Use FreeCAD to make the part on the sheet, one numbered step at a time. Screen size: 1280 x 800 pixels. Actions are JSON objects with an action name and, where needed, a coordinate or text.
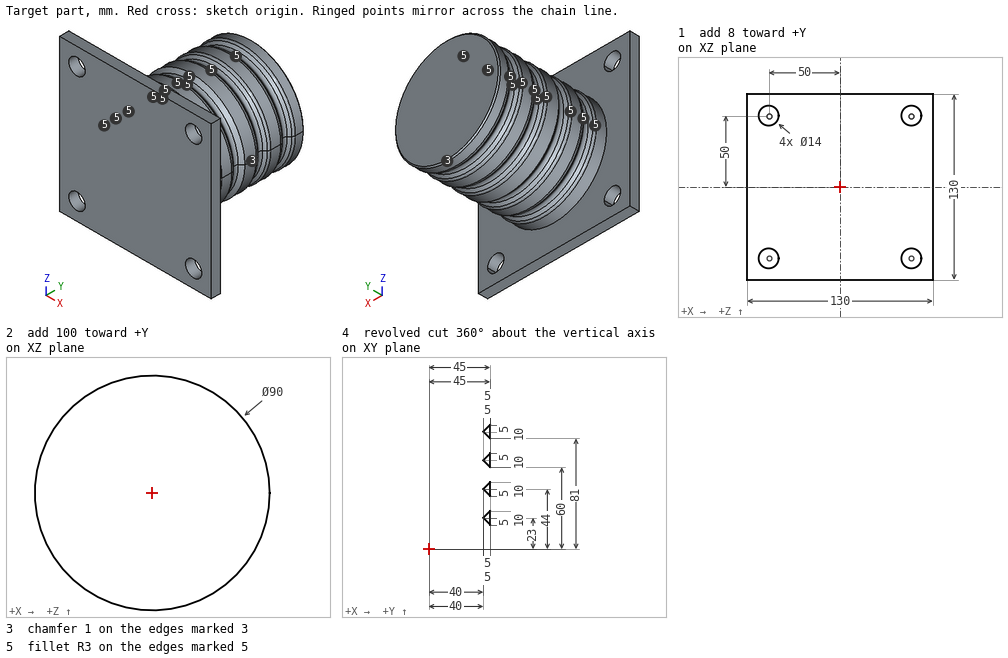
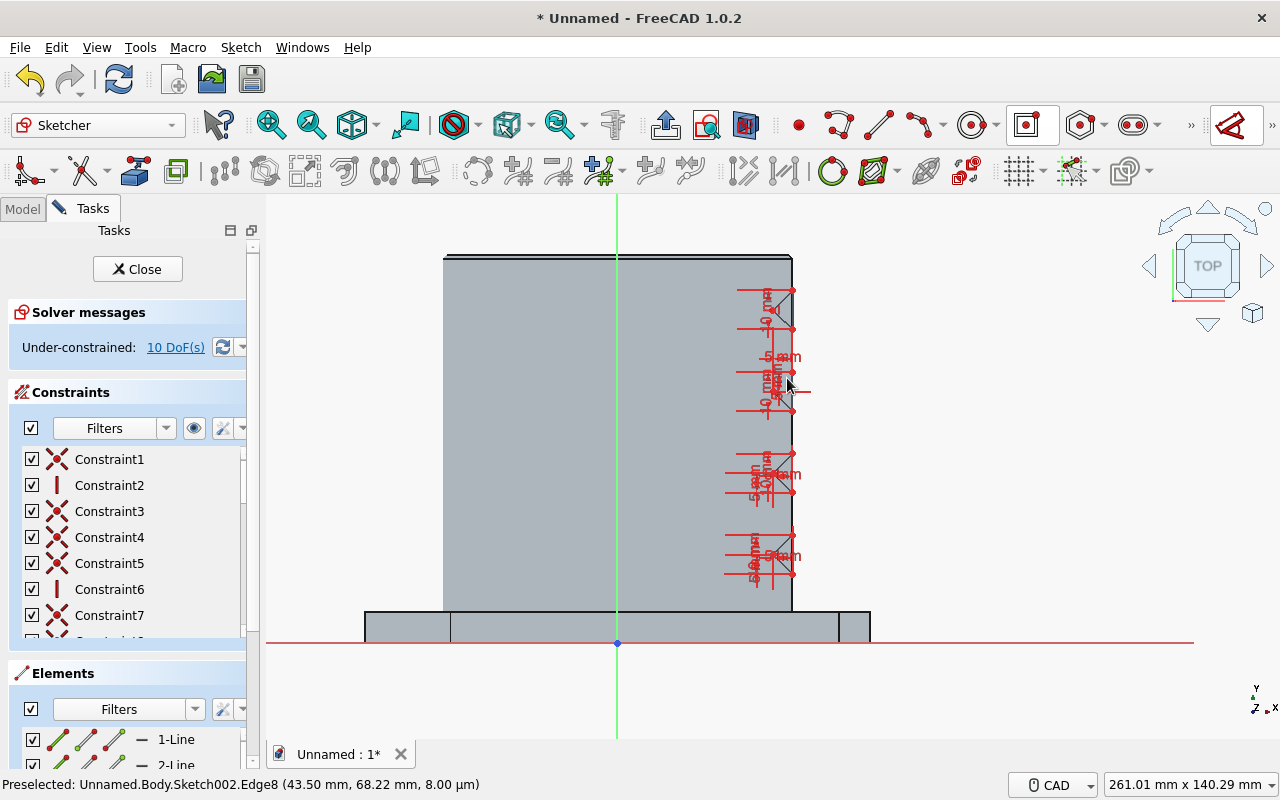
{"action": "scroll", "coordinate": [787, 296], "scroll_direction": "up", "scroll_amount": 5}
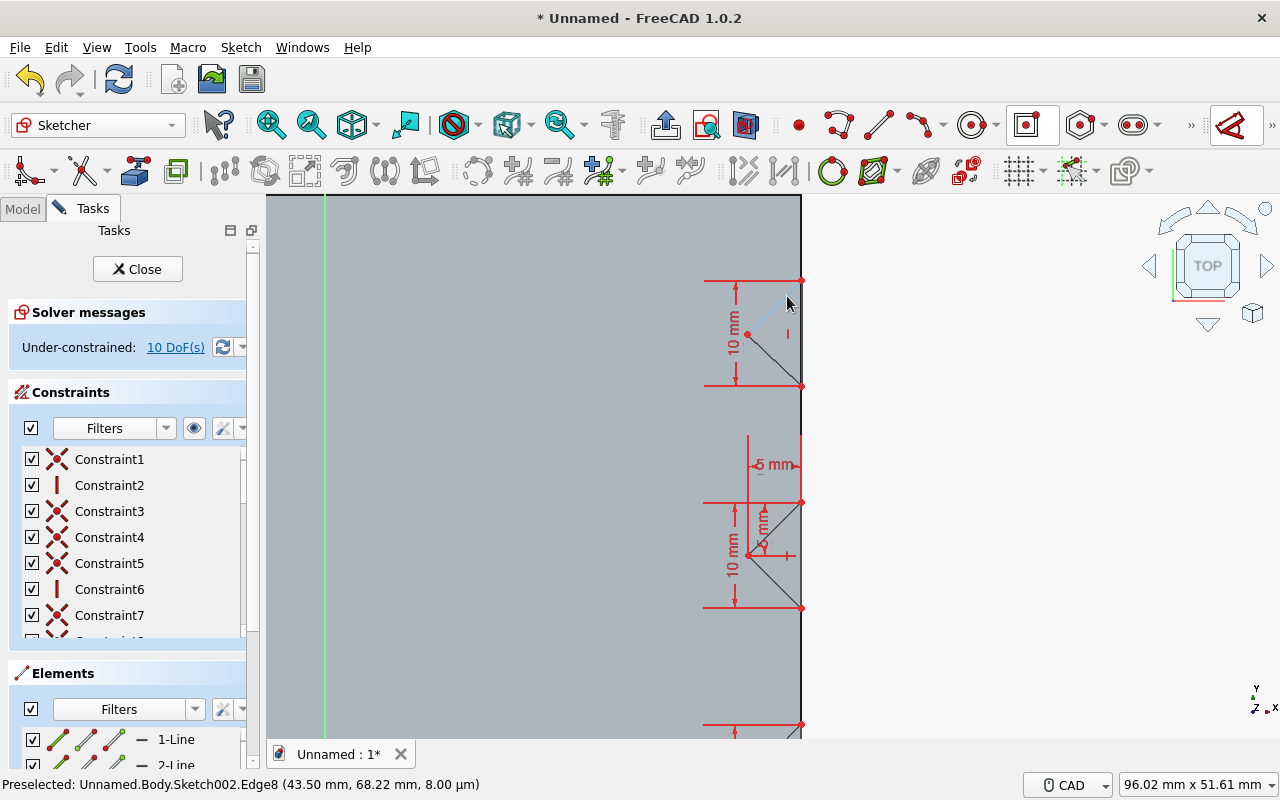
{"action": "left_click", "coordinate": [786, 297]}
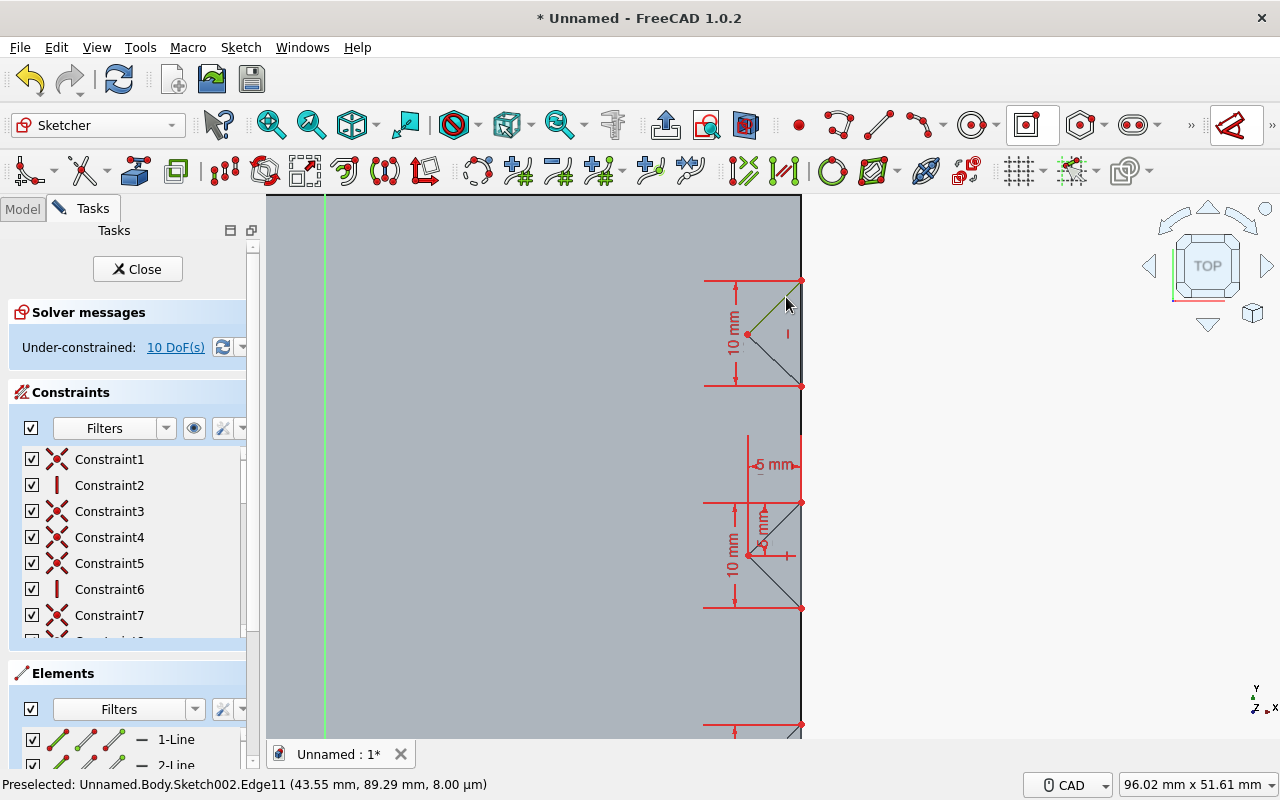
{"action": "key", "text": "l"}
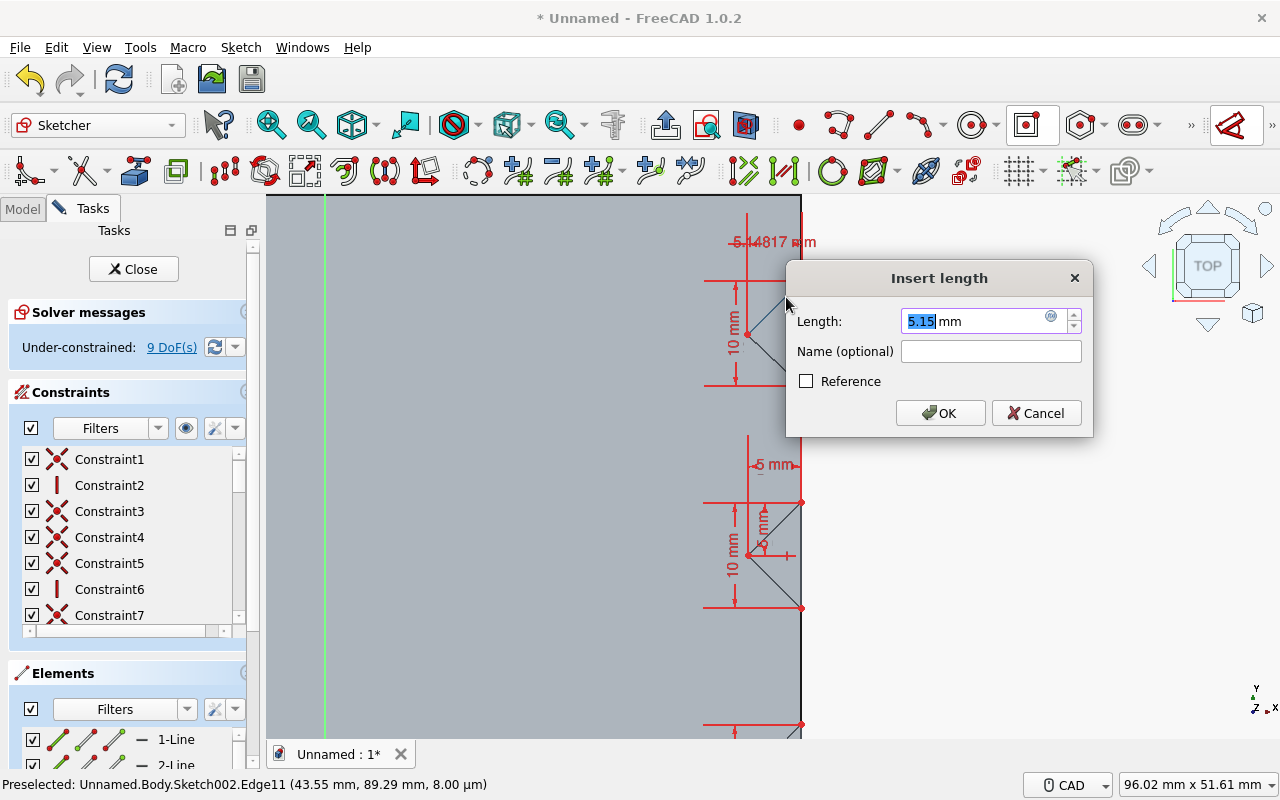
{"action": "type", "text": "5"}
{"action": "key", "text": "Return"}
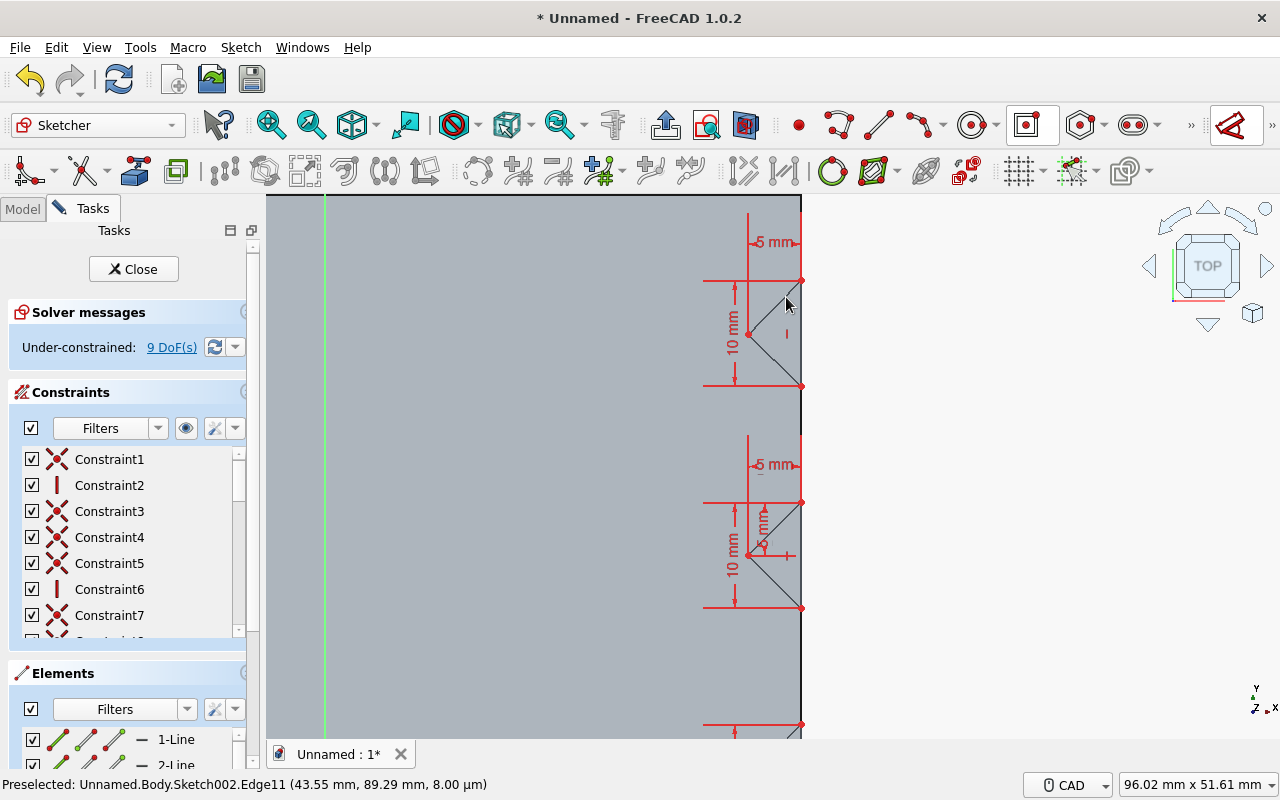
{"action": "left_click", "coordinate": [785, 297]}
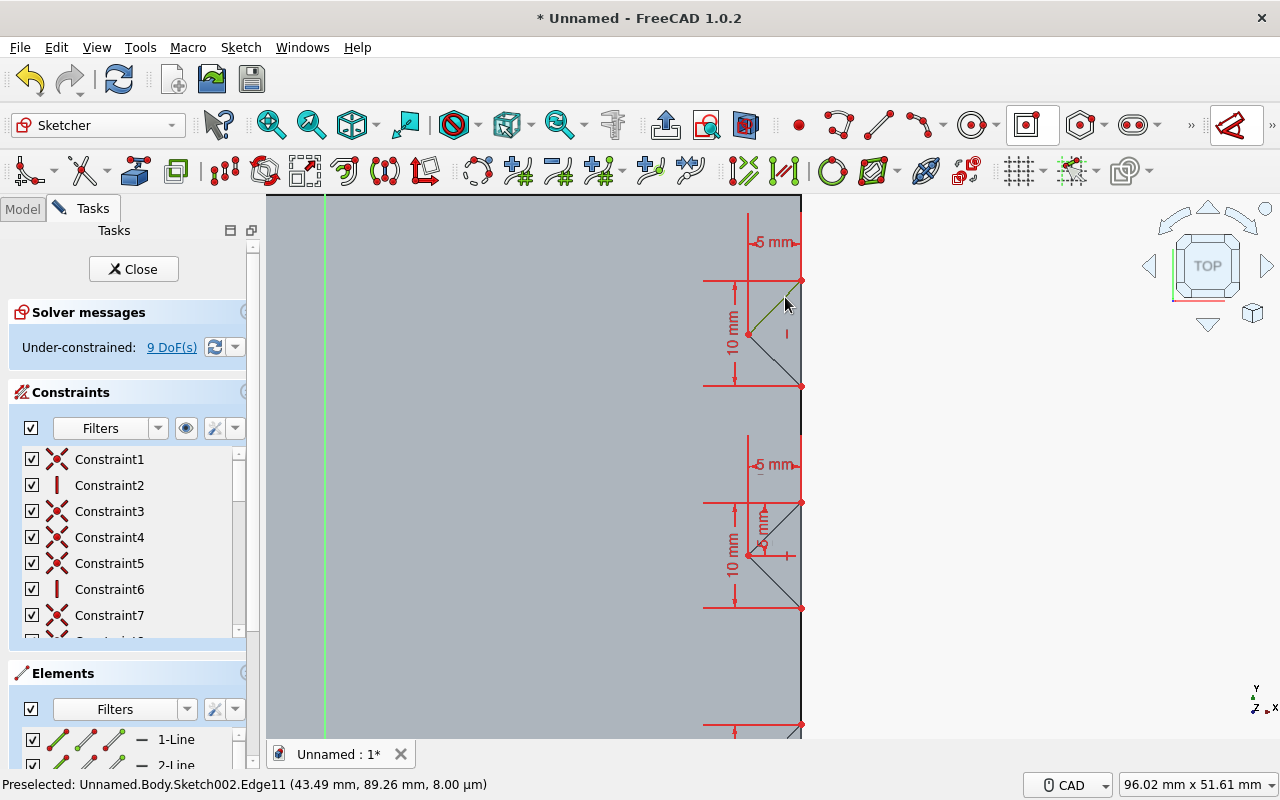
{"action": "left_click", "coordinate": [1258, 126]}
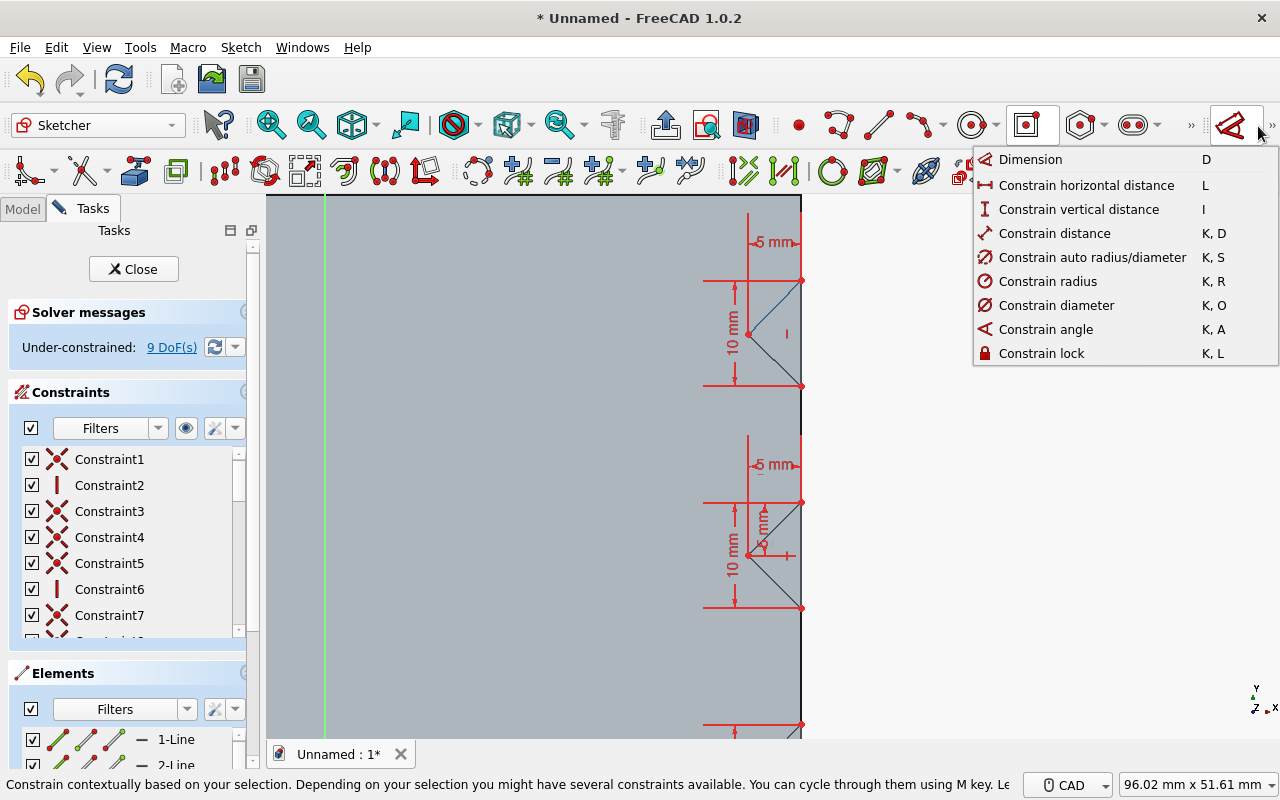
{"action": "left_click", "coordinate": [1126, 209]}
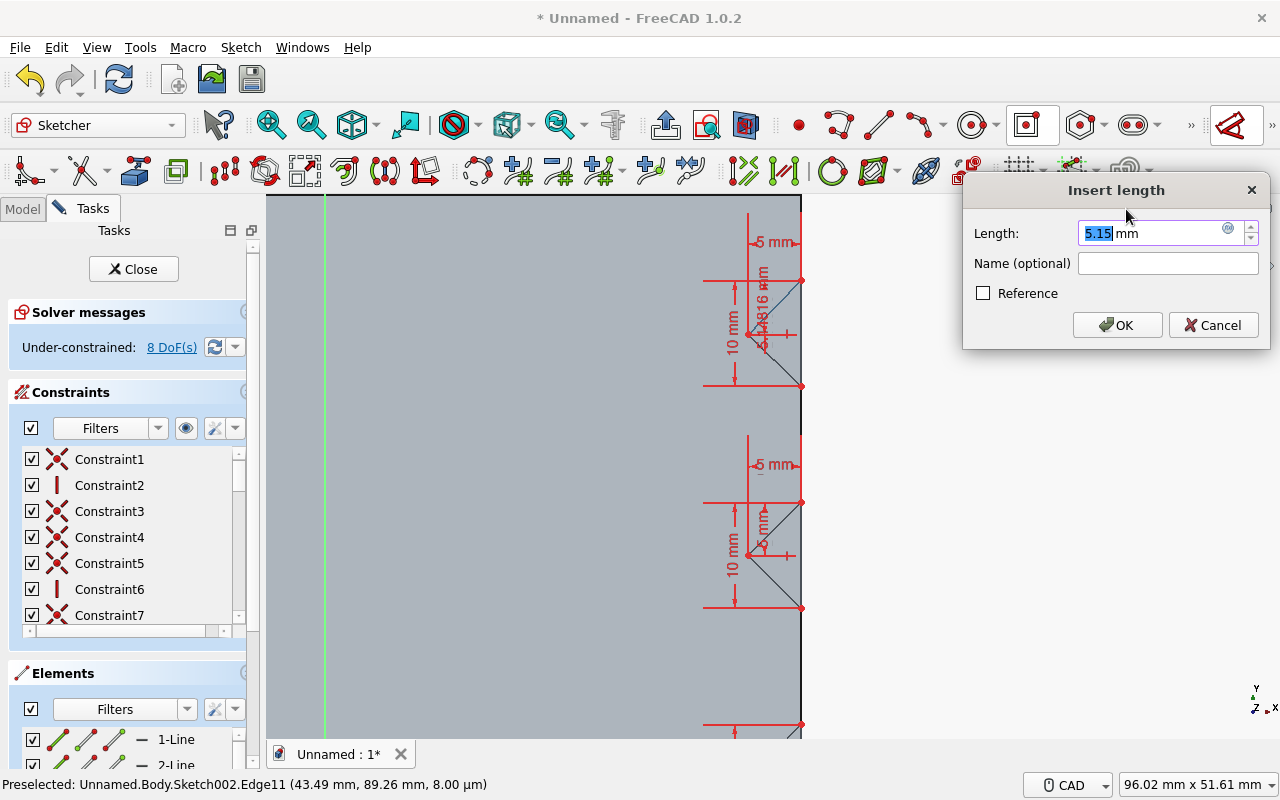
{"action": "type", "text": "5"}
{"action": "key", "text": "Return"}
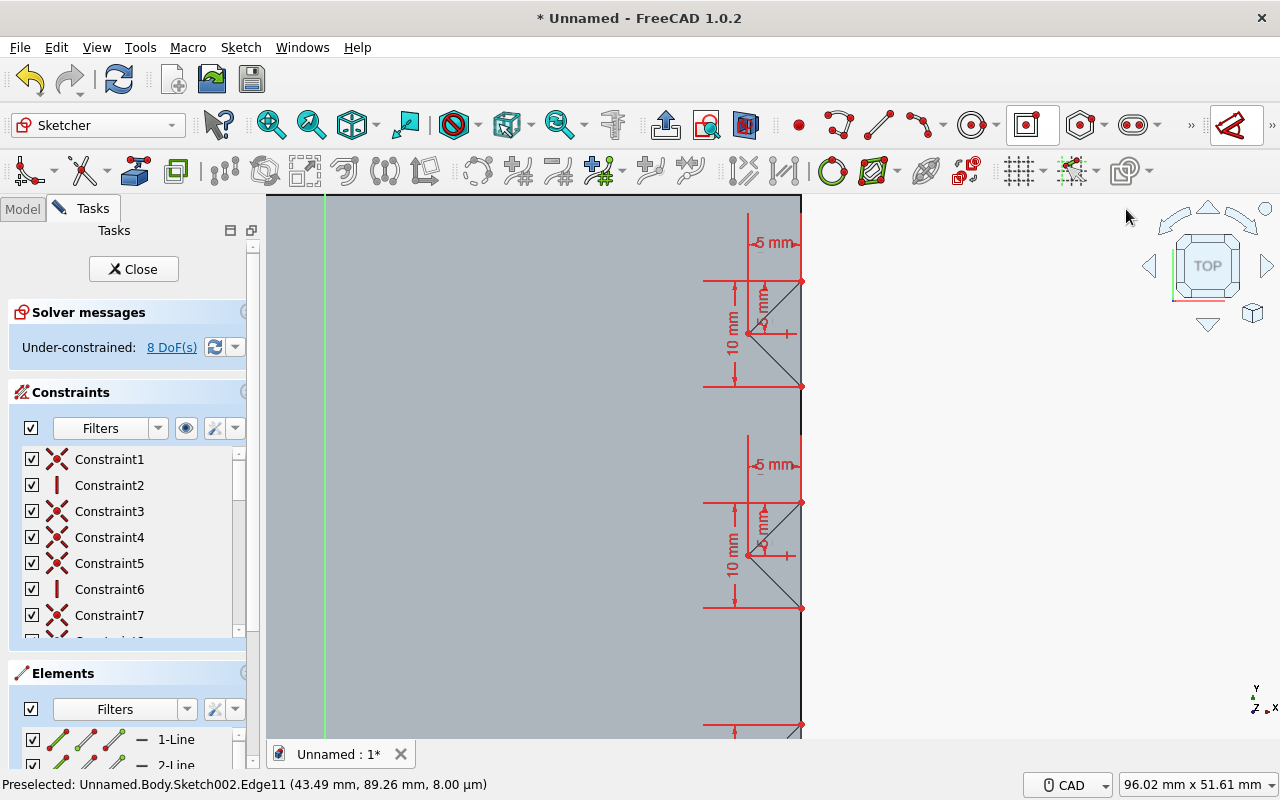
{"action": "scroll", "coordinate": [787, 296], "scroll_direction": "down", "scroll_amount": 5}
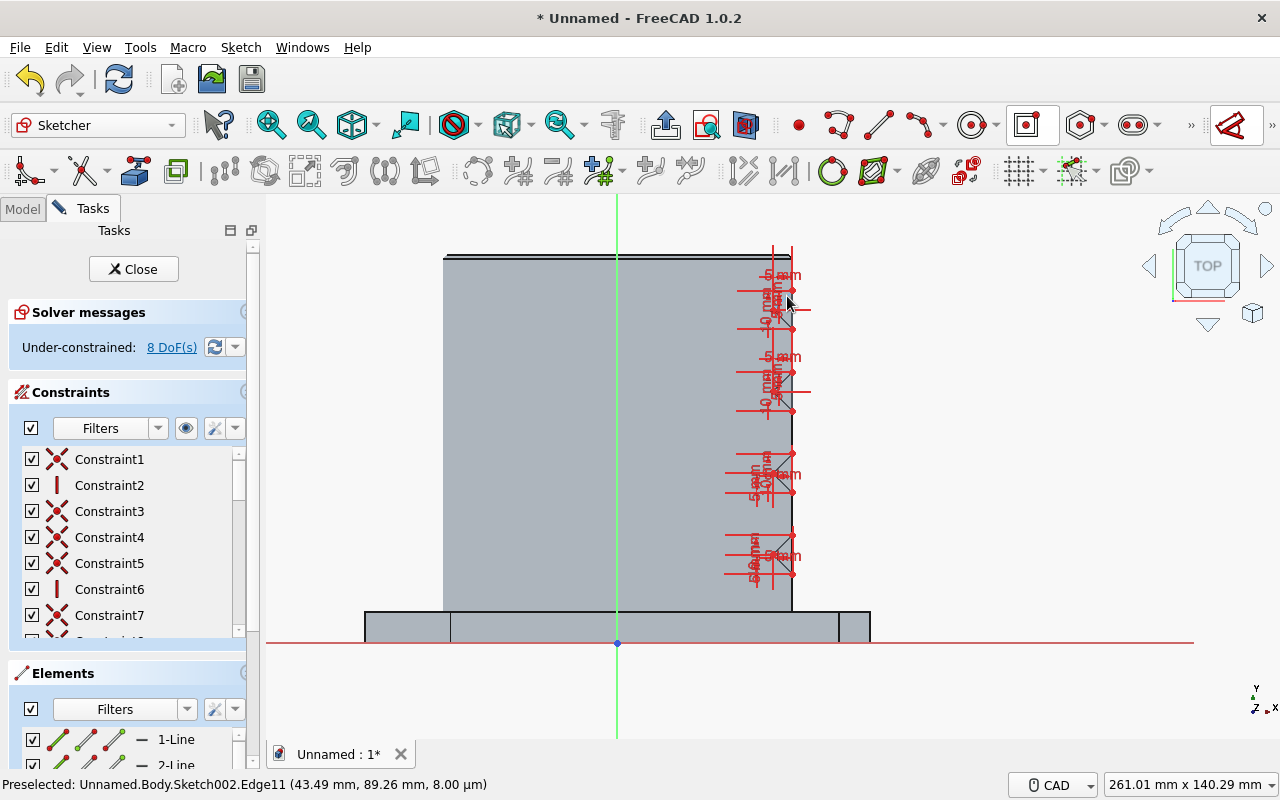
{"action": "left_click", "coordinate": [773, 555]}